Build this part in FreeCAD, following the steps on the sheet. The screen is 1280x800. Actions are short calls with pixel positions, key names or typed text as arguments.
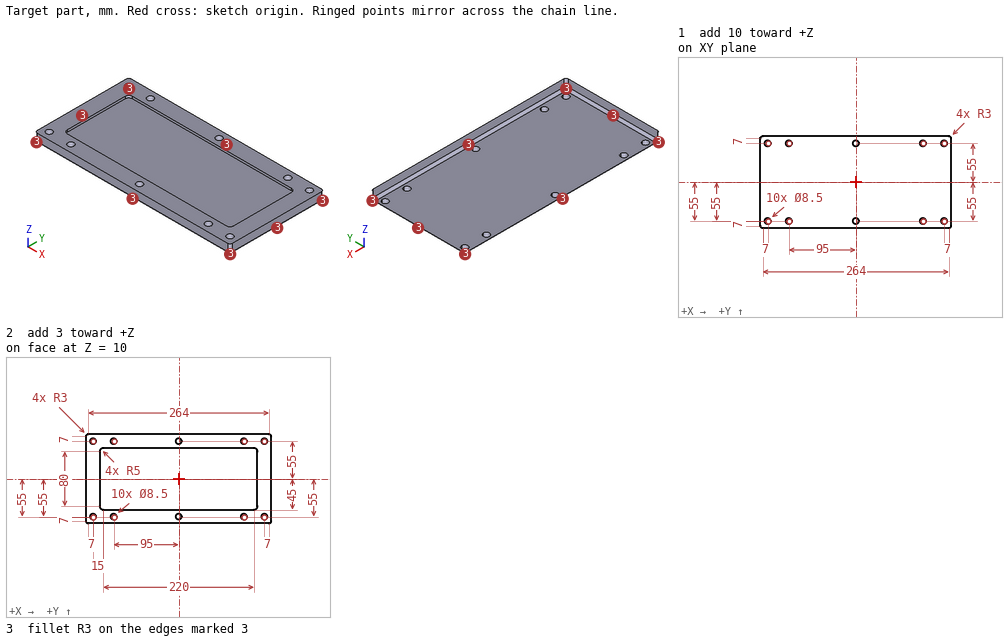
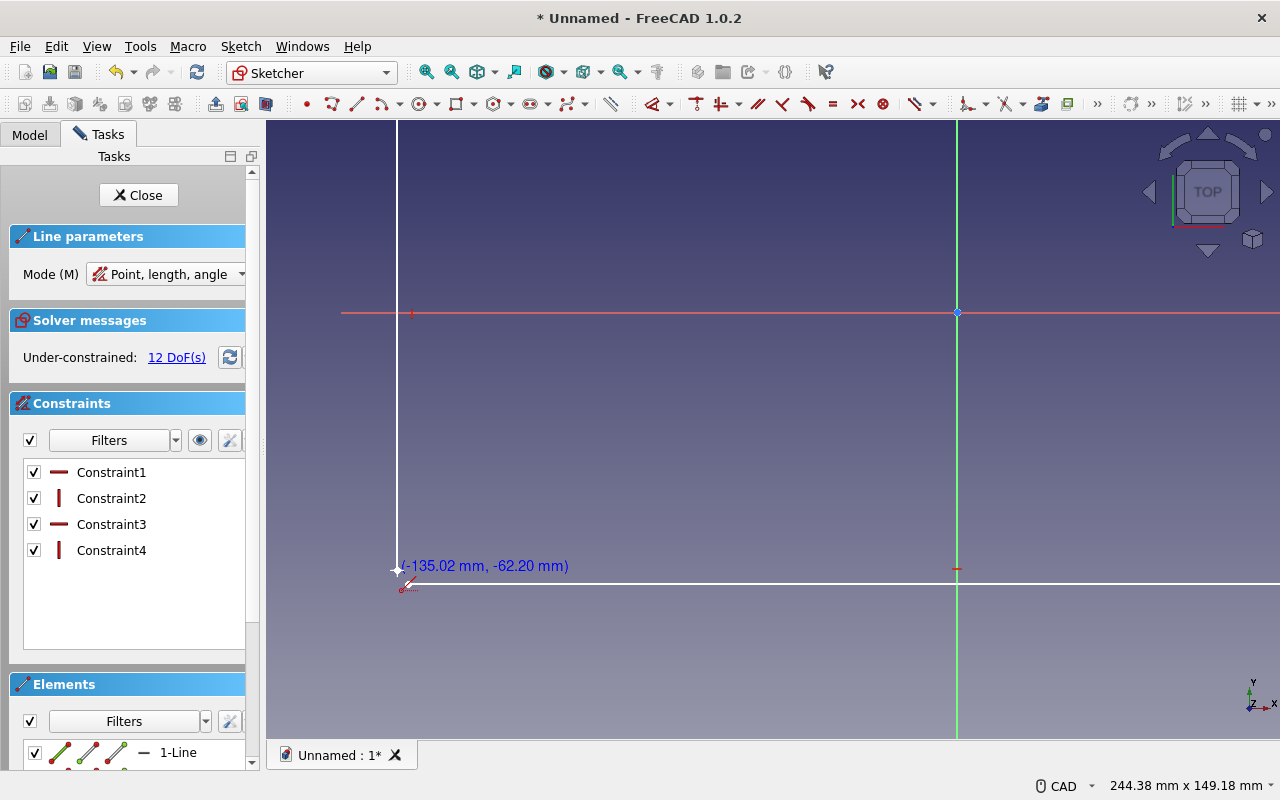
click(400, 104)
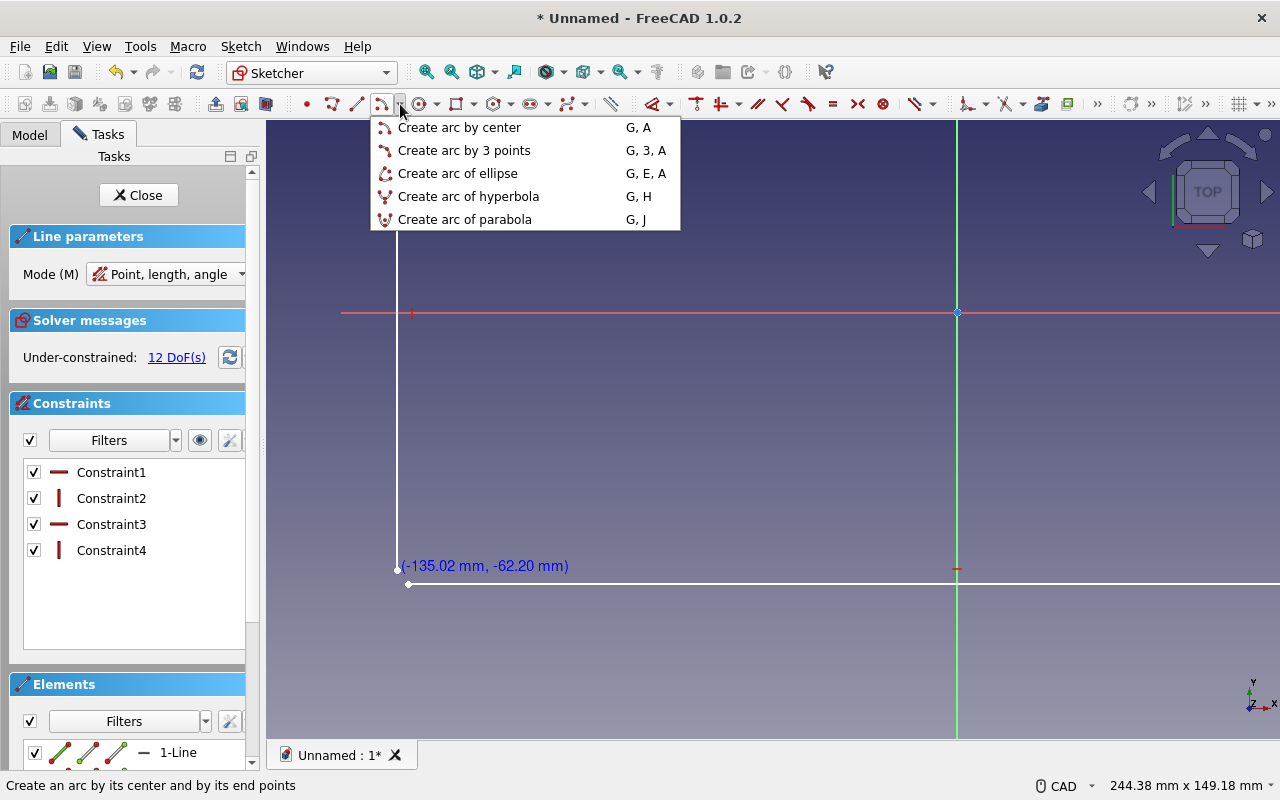
click(526, 150)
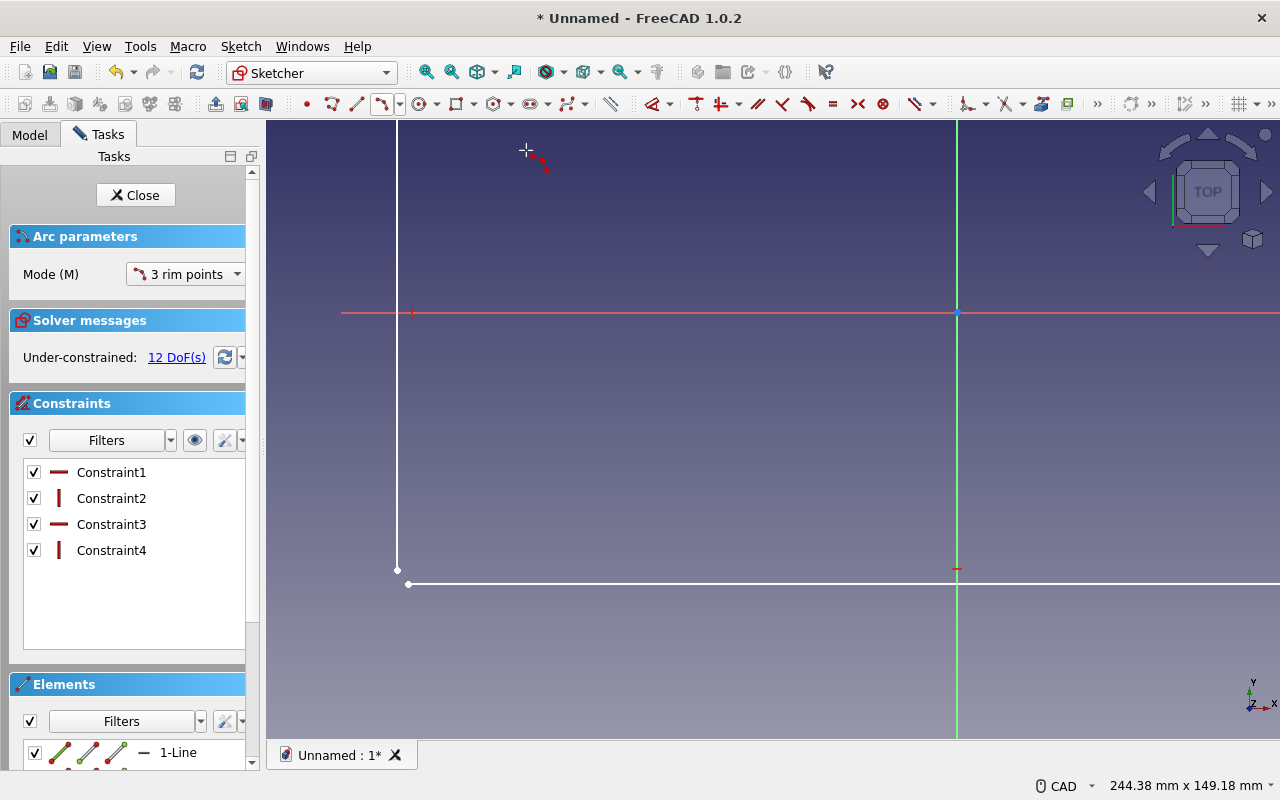
scroll(397, 571, down, 3)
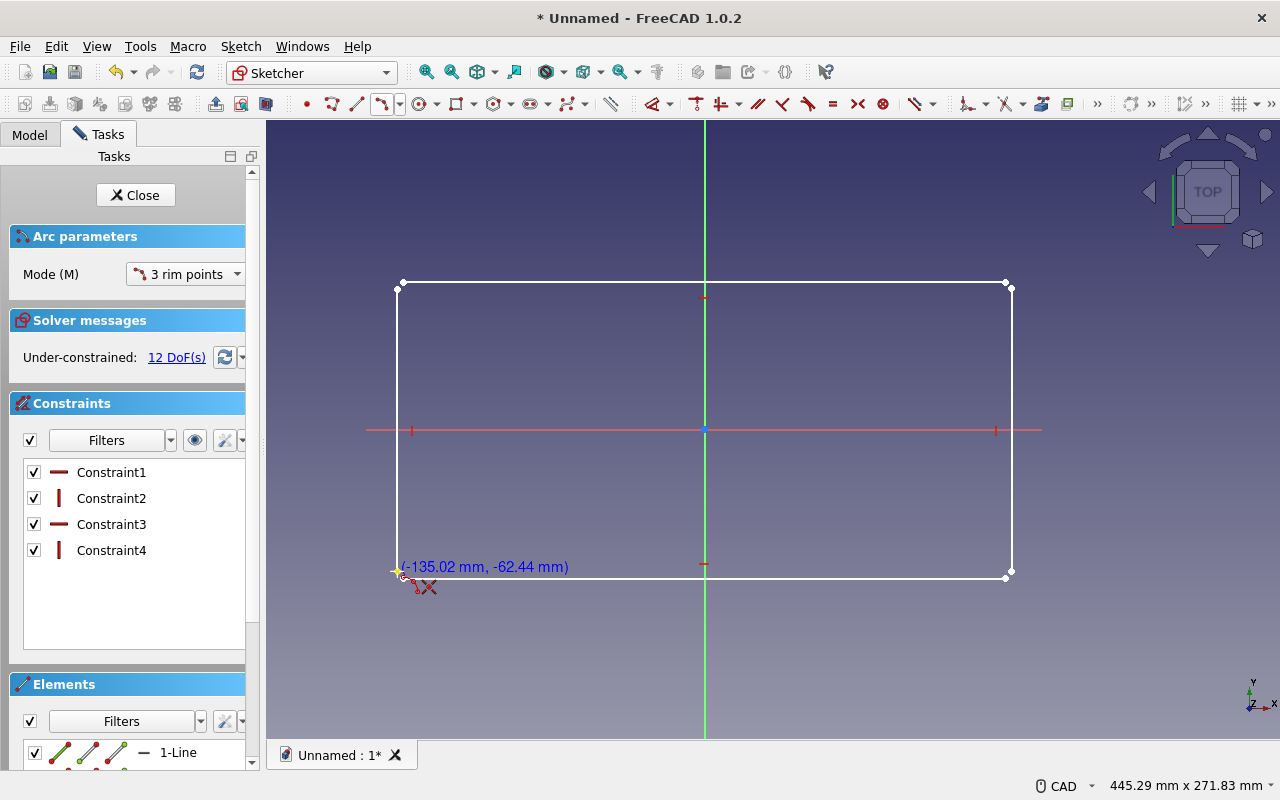
scroll(1005, 578, up, 3)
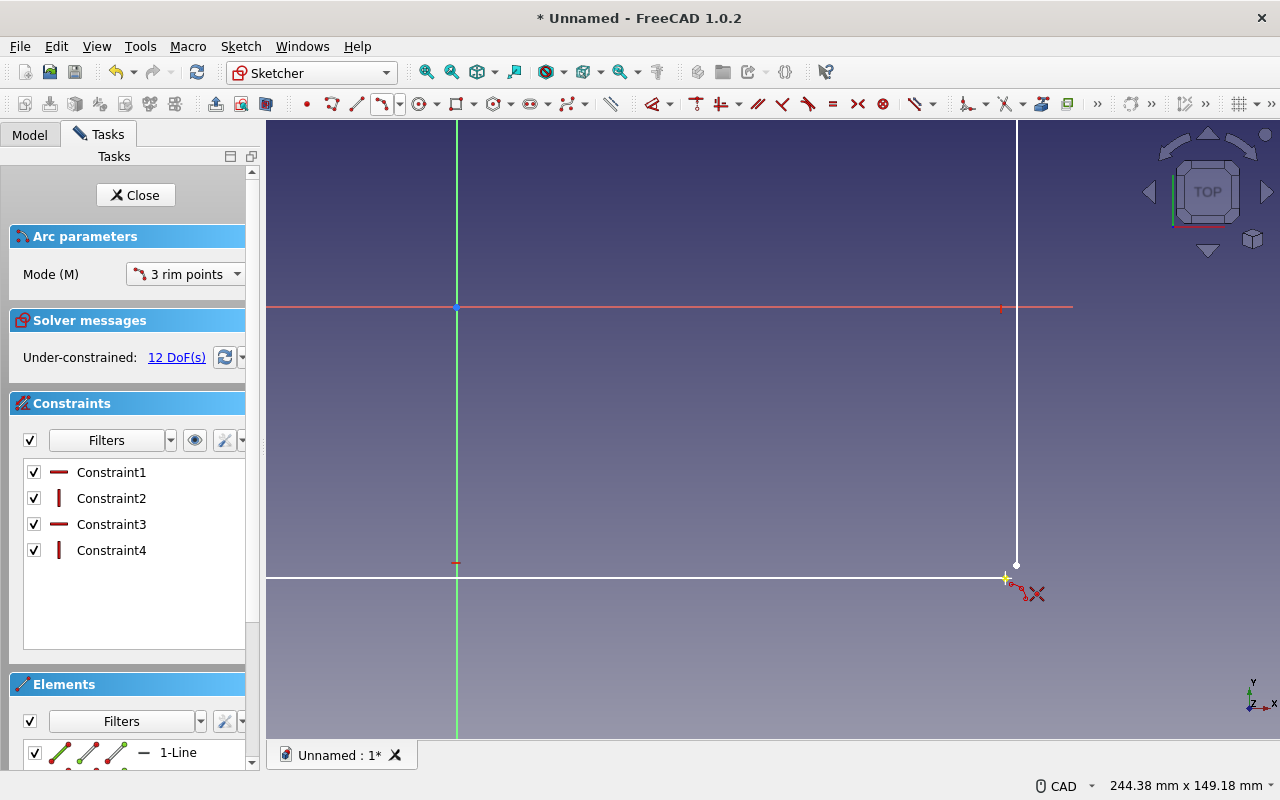
click(1005, 578)
click(1017, 565)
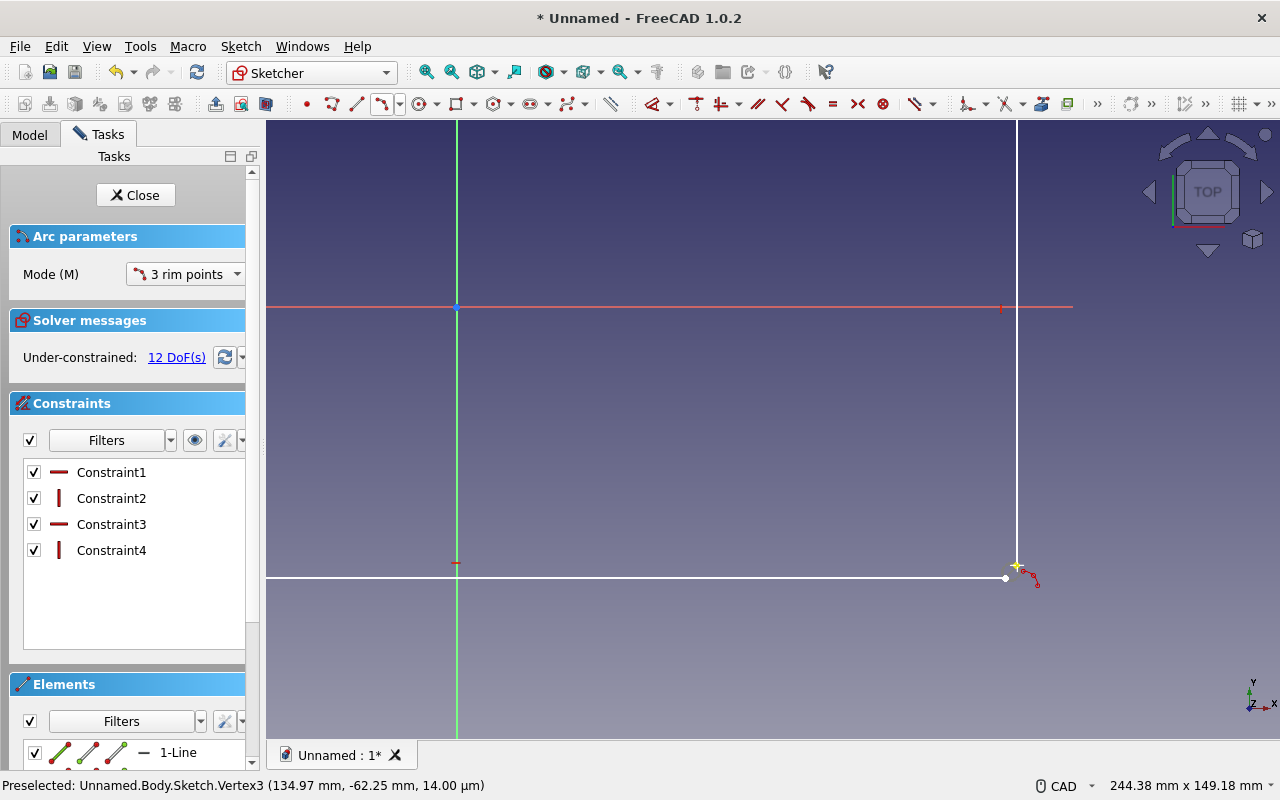
scroll(1013, 573, up, 8)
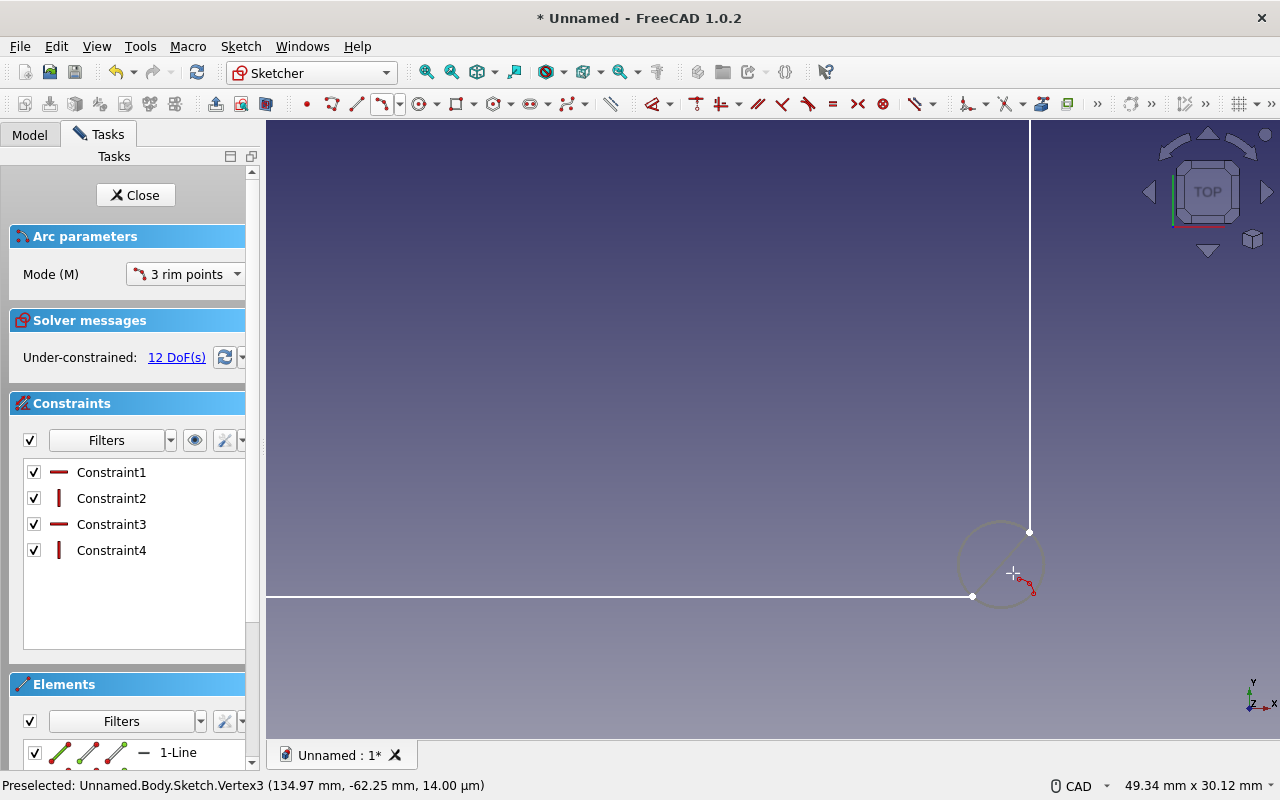
click(1012, 571)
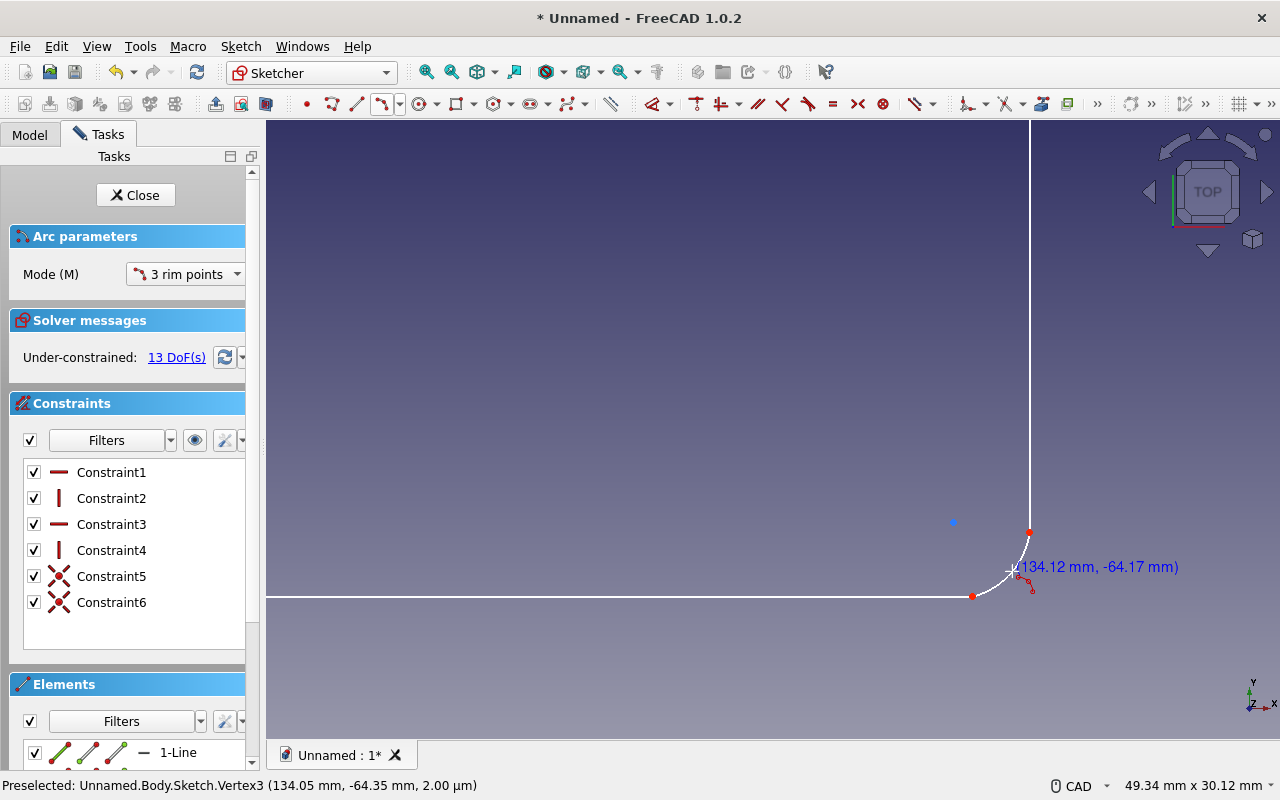
scroll(1010, 576, down, 11)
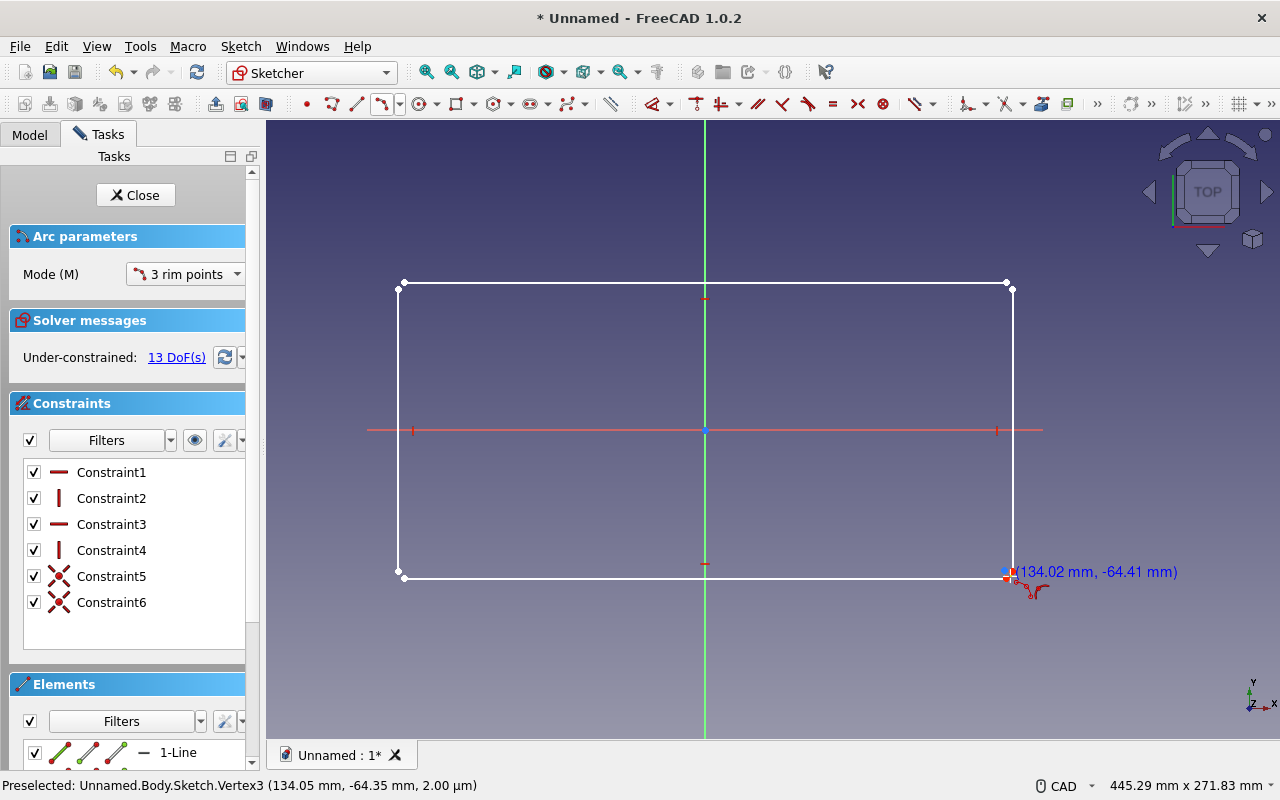
scroll(1013, 289, up, 3)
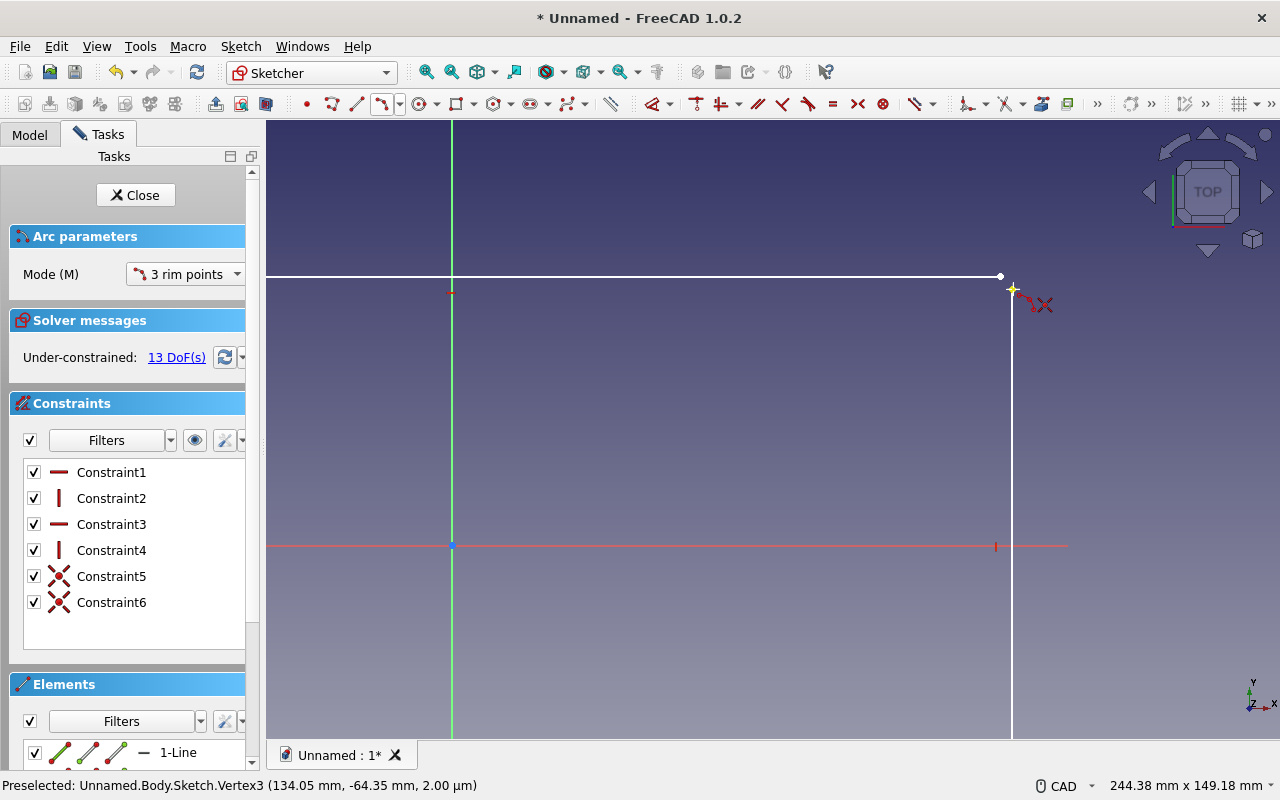
click(1012, 290)
click(1000, 277)